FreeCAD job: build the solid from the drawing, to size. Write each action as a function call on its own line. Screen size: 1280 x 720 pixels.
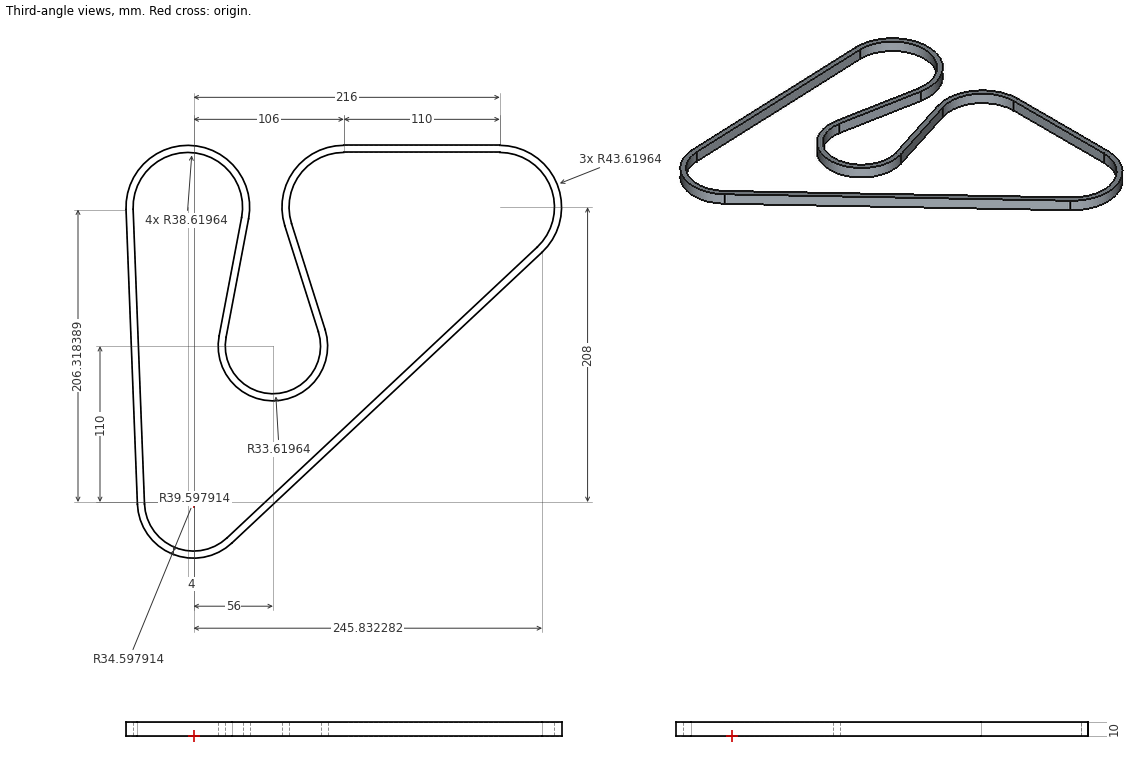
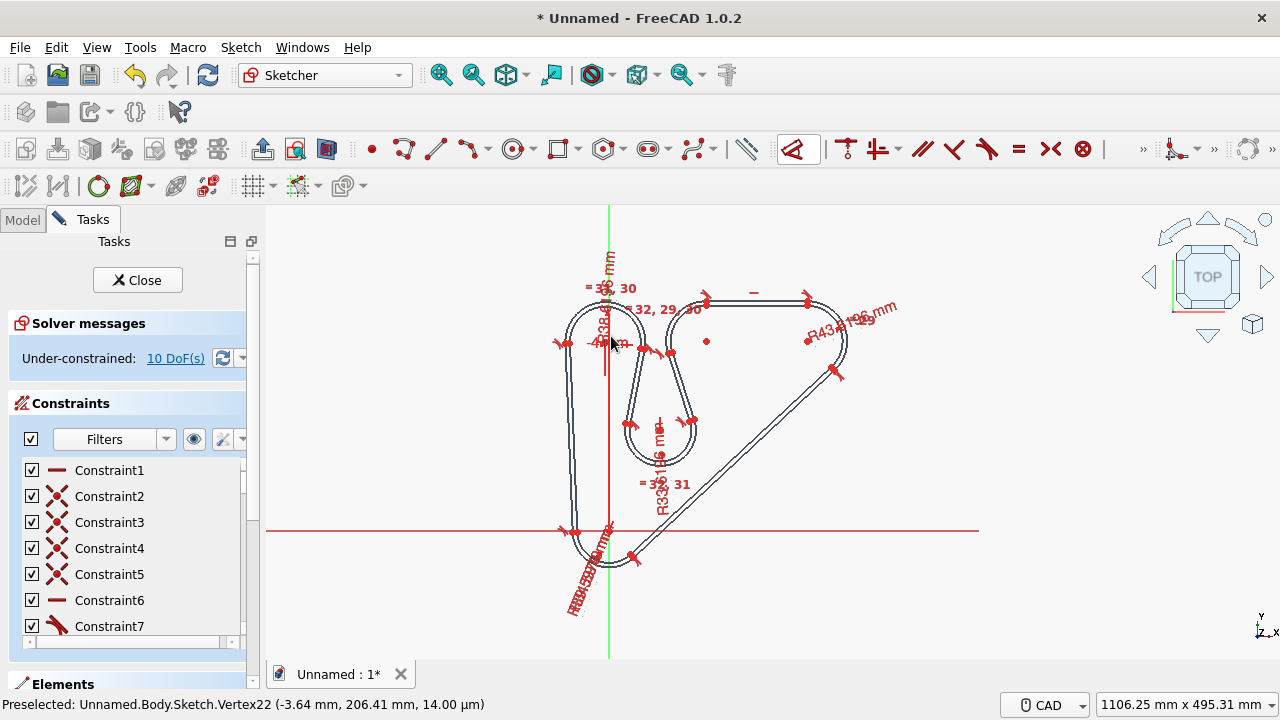
scroll(777, 301, up, 6)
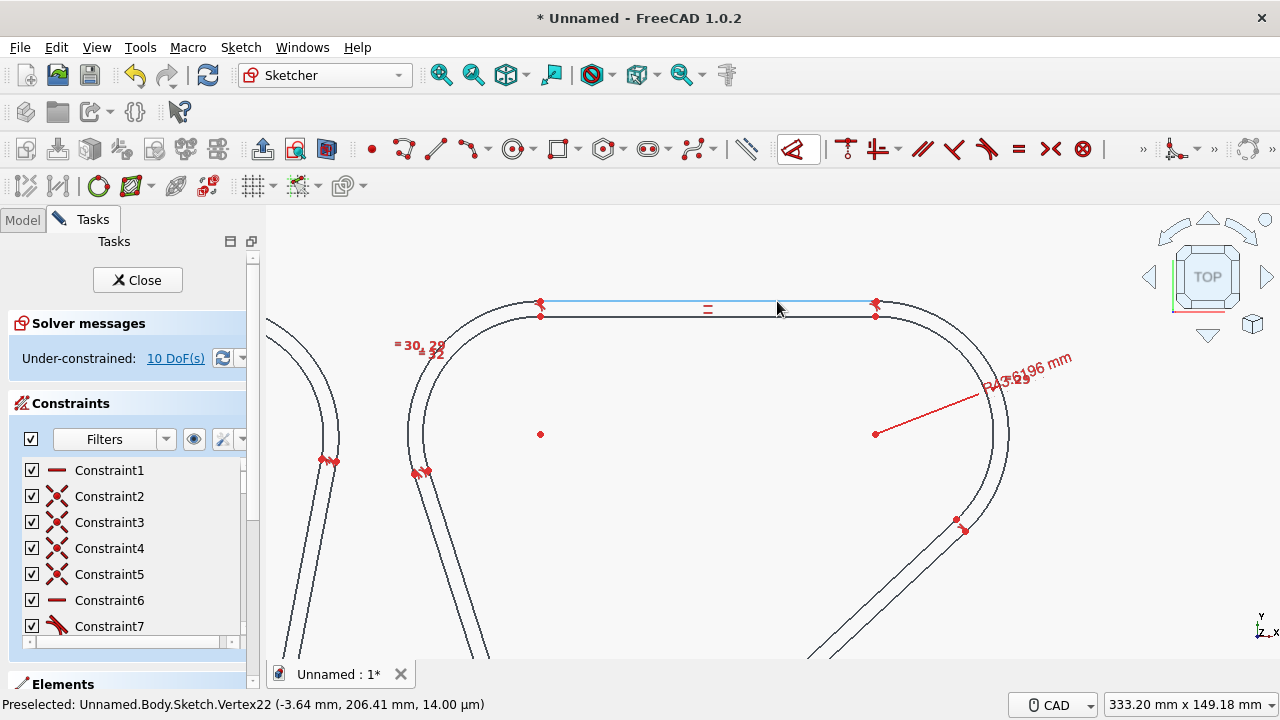
click(775, 301)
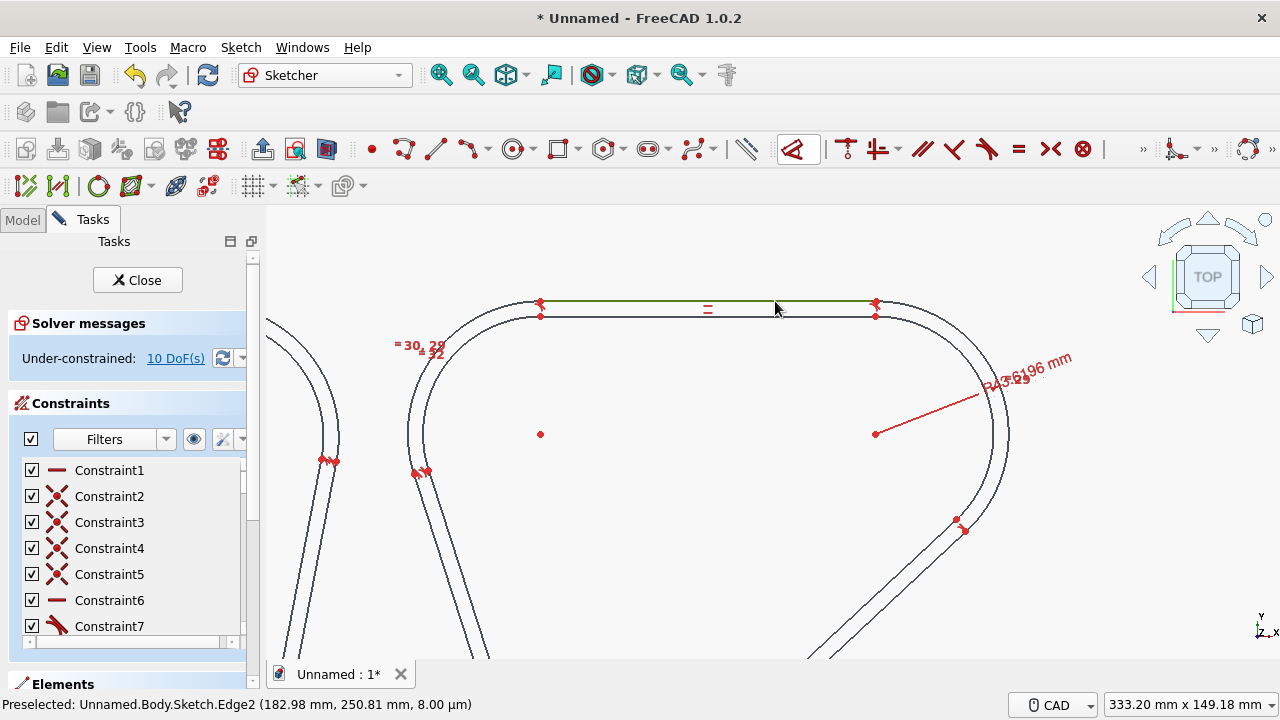
key(l)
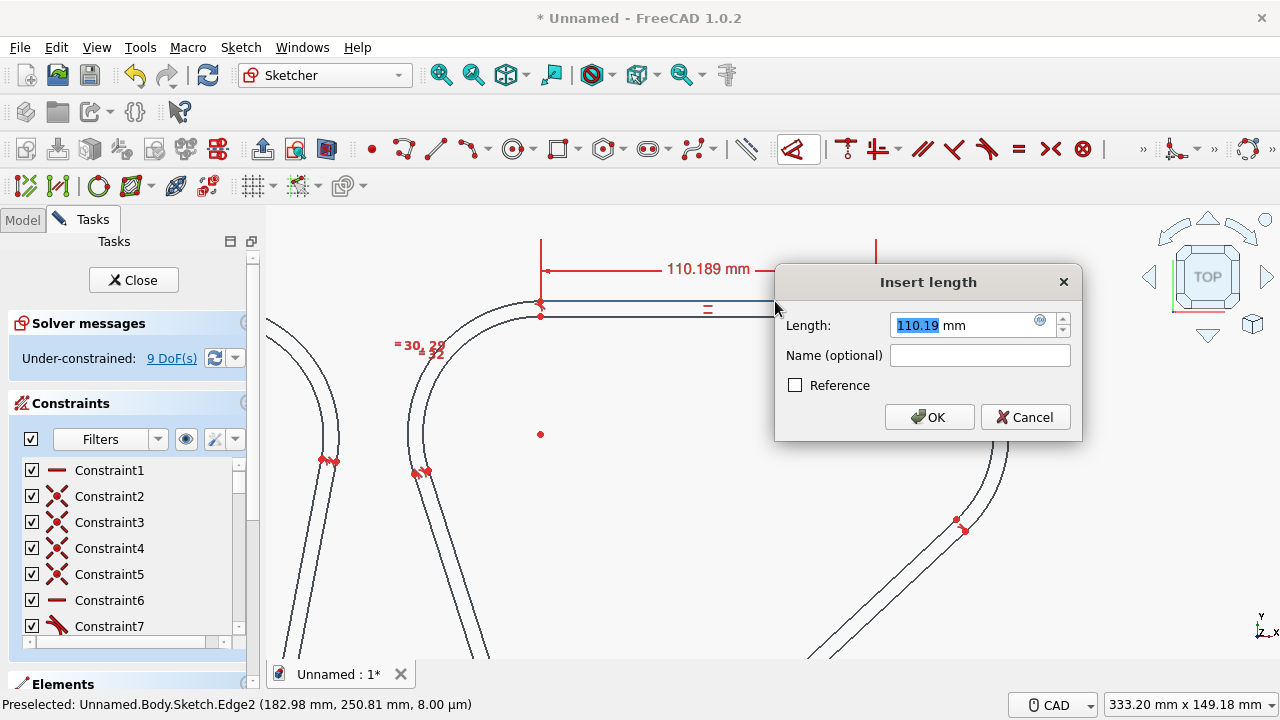
text(110)
key(Return)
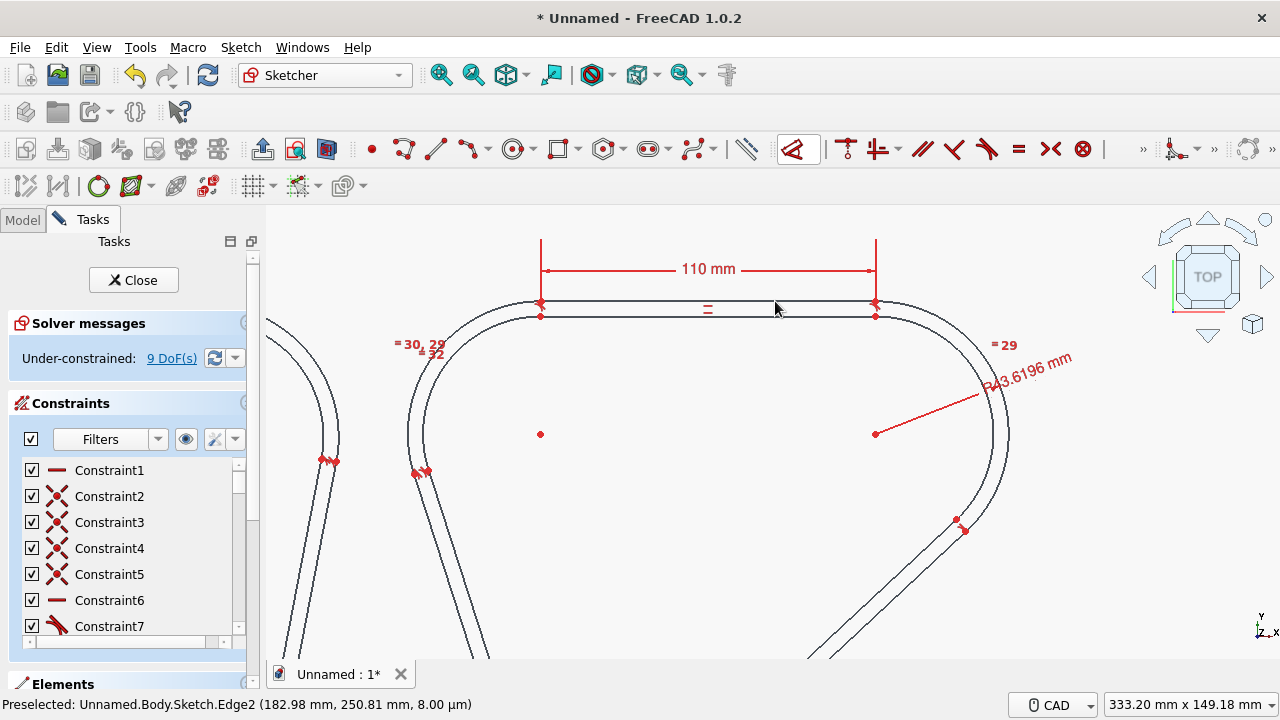
click(641, 317)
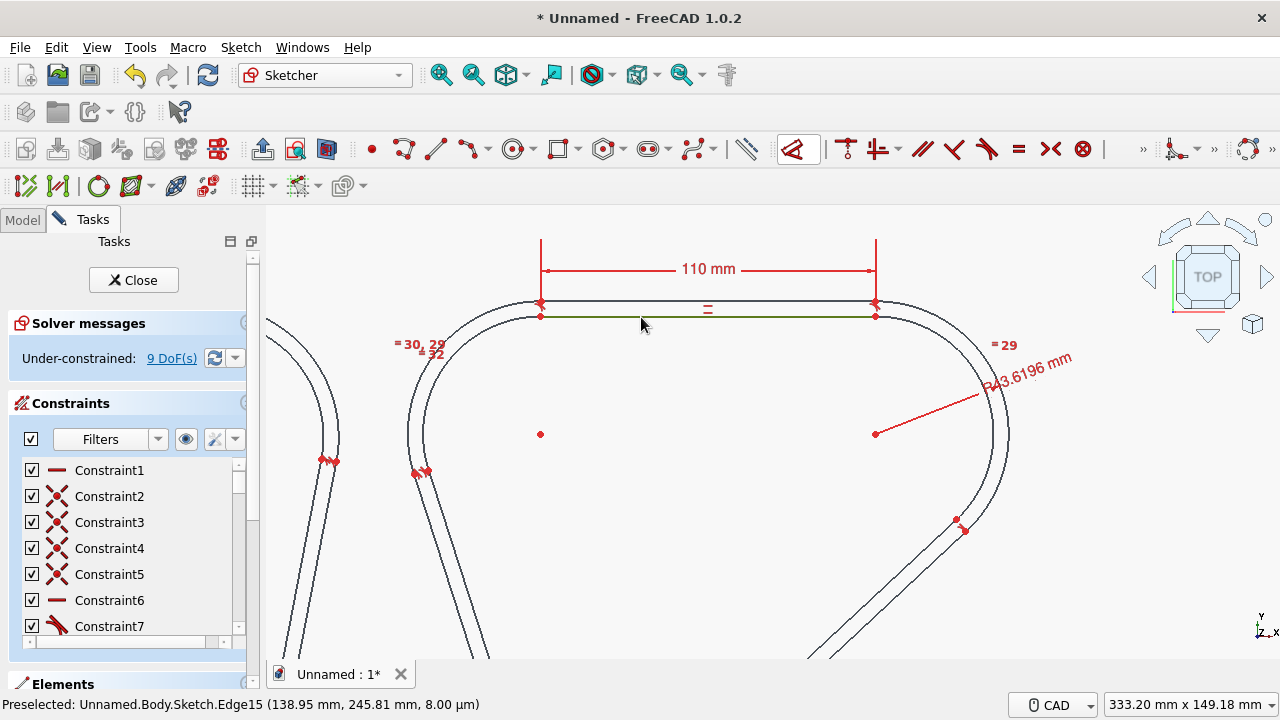
key(l)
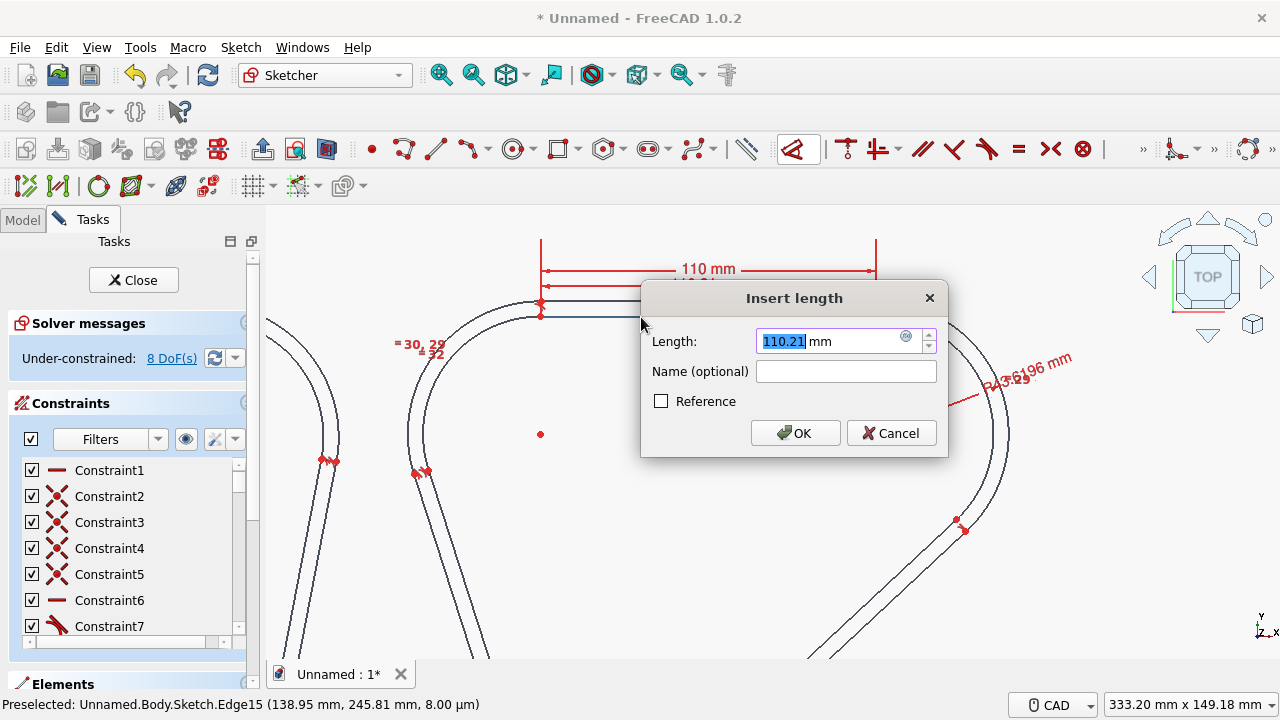
text(110)
key(Return)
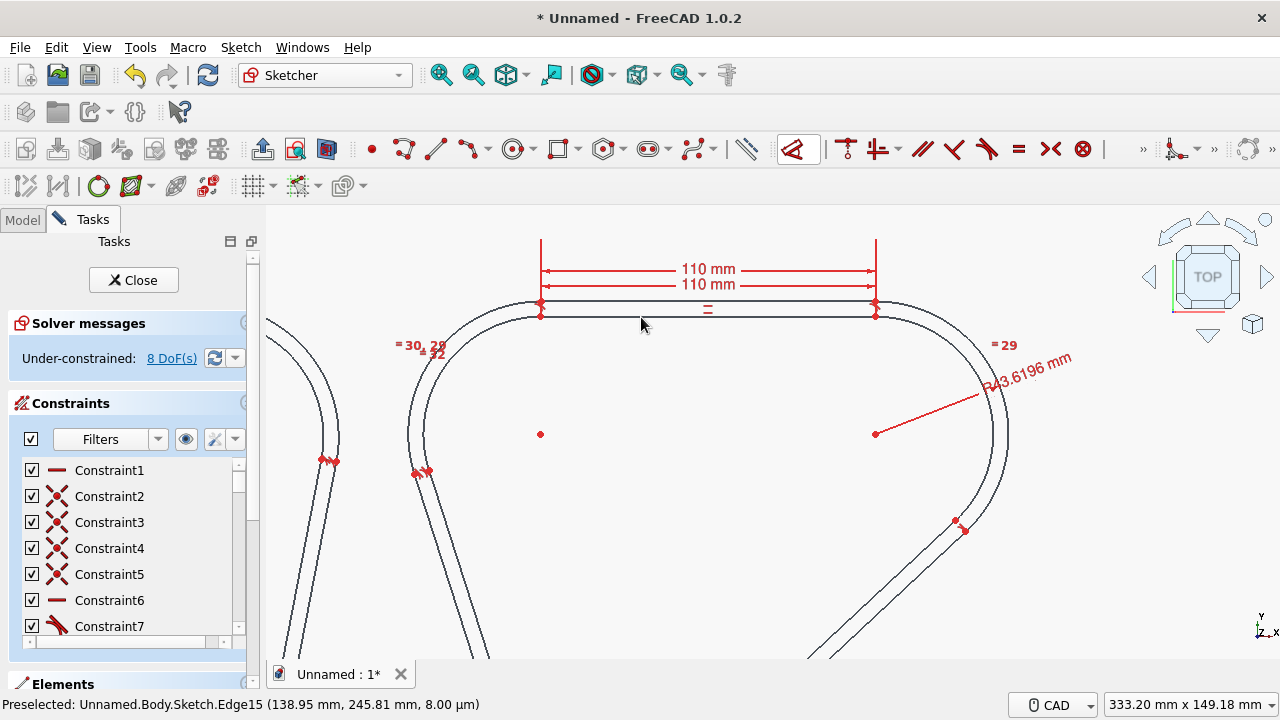
scroll(777, 300, down, 6)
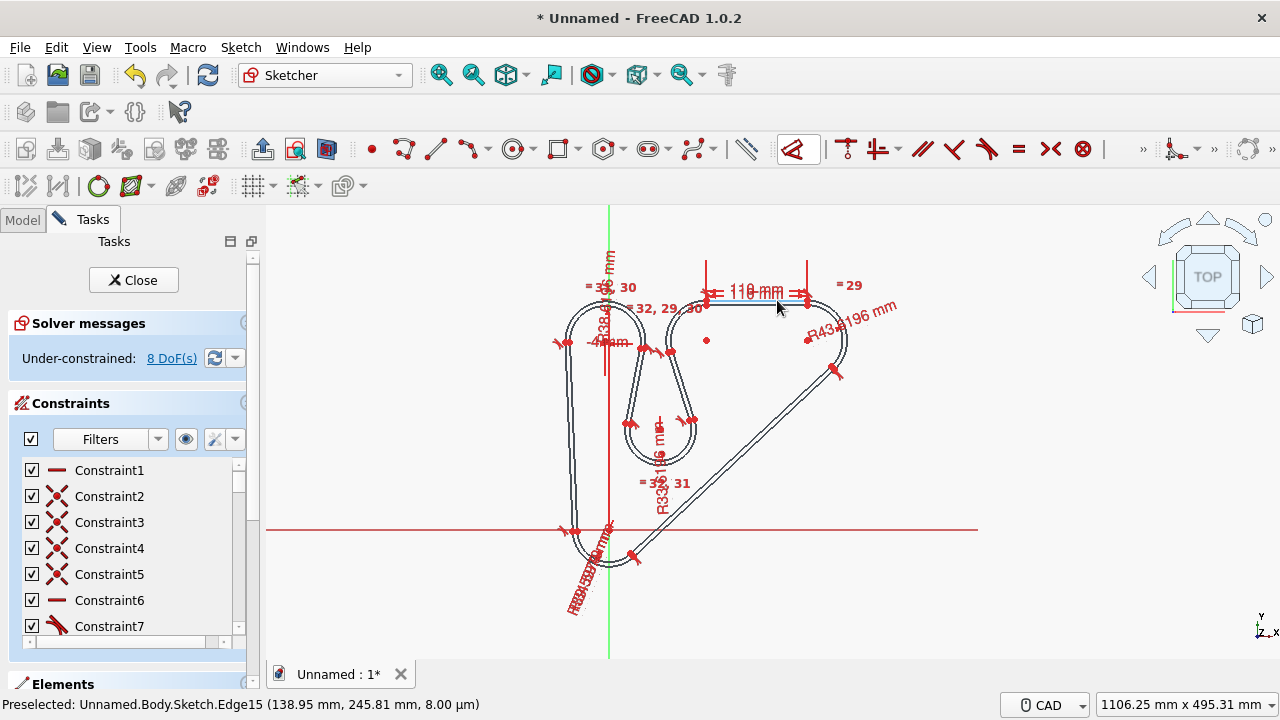
click(660, 430)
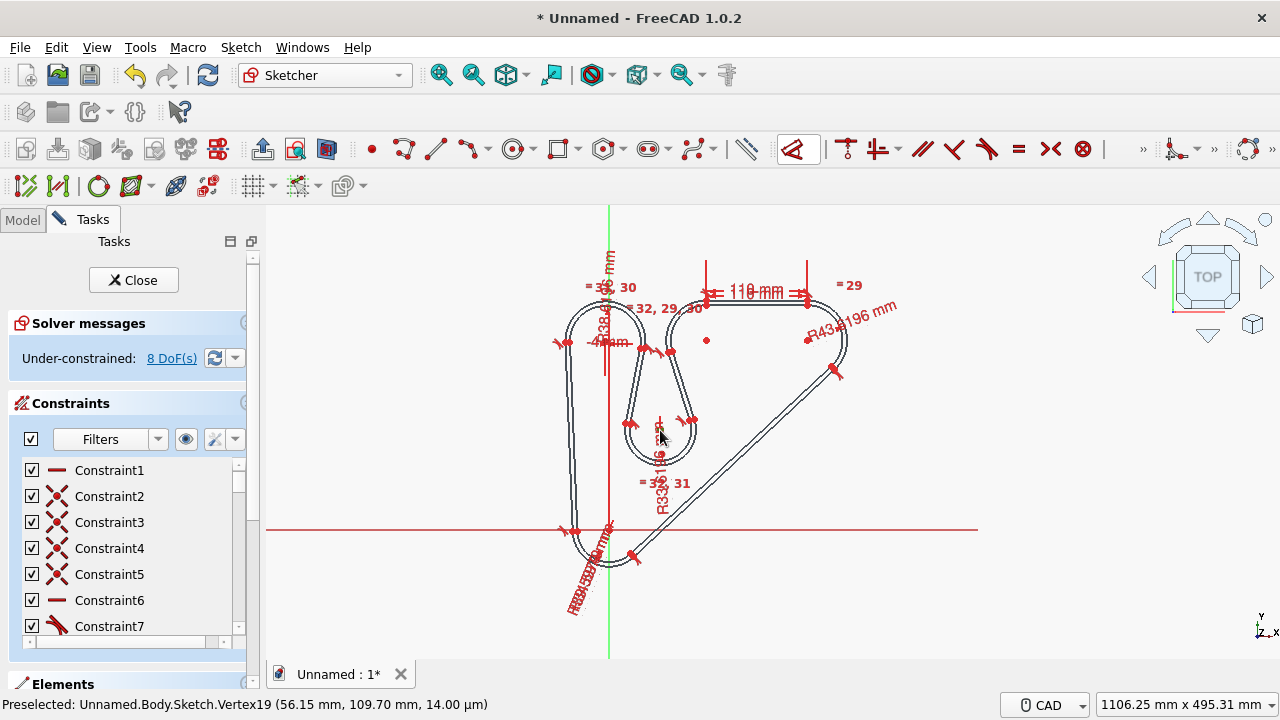
key(l)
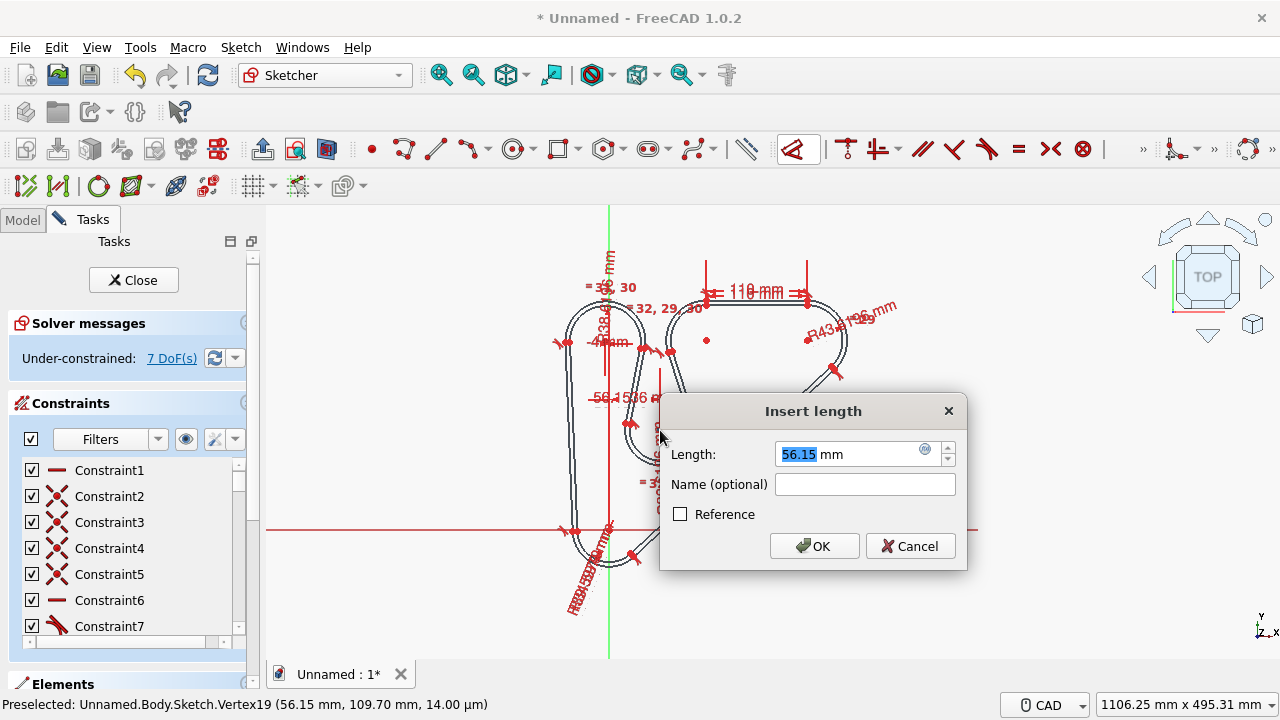
text(56)
key(Return)